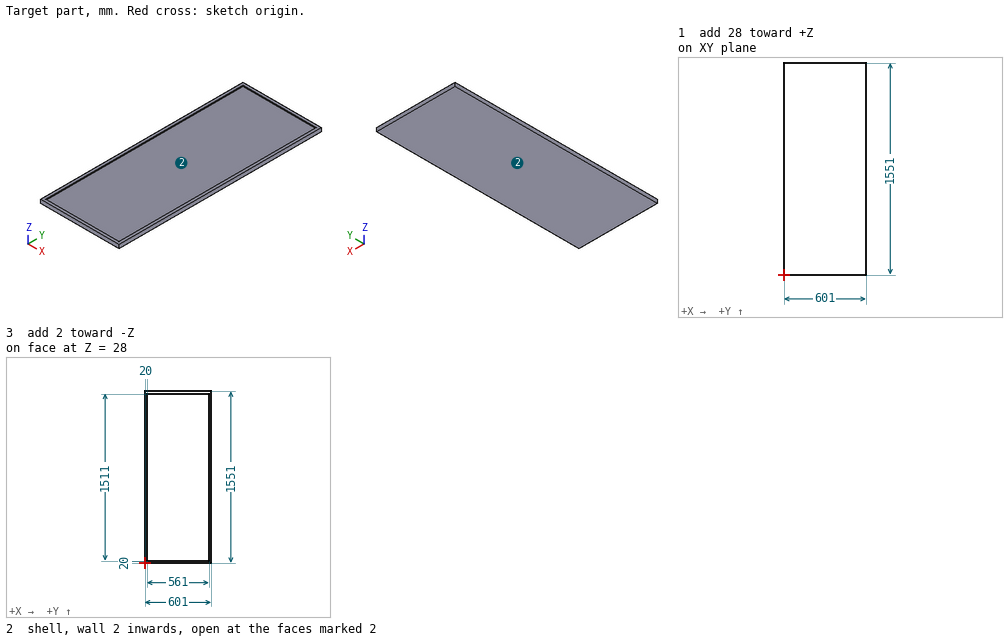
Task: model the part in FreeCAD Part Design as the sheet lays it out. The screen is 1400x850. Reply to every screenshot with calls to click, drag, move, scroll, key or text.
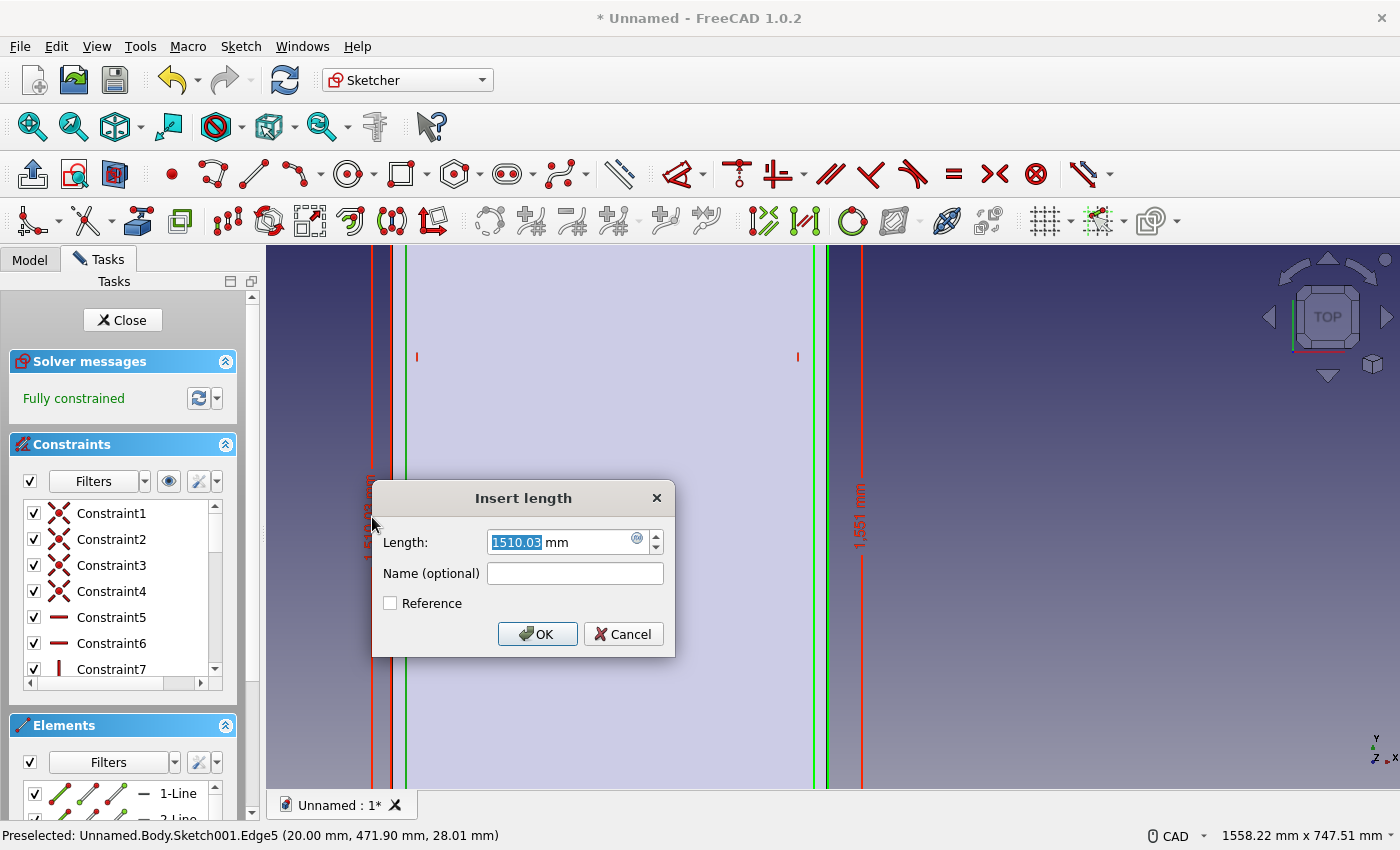
text(1511)
key(Return)
key(Escape)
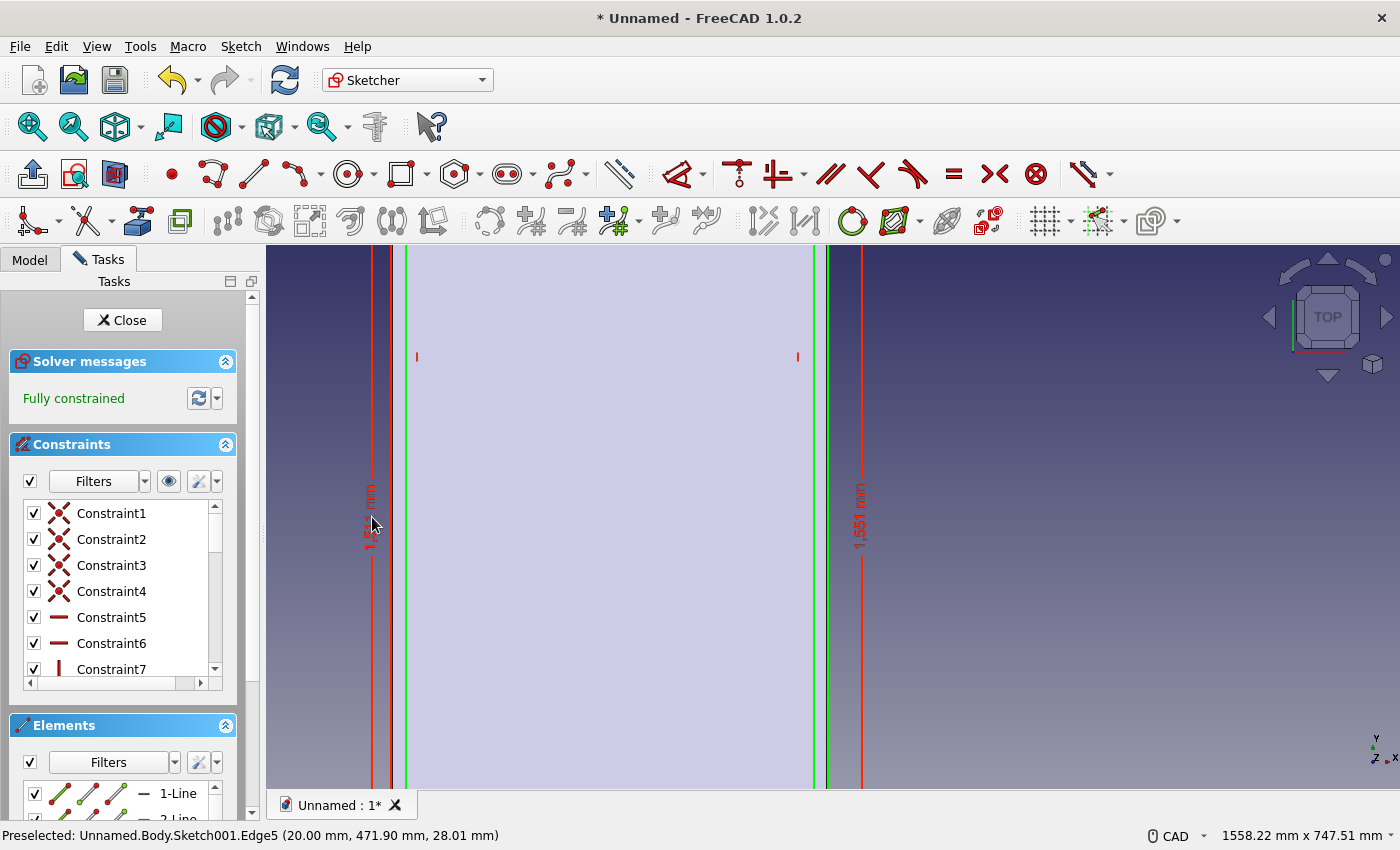
click(123, 320)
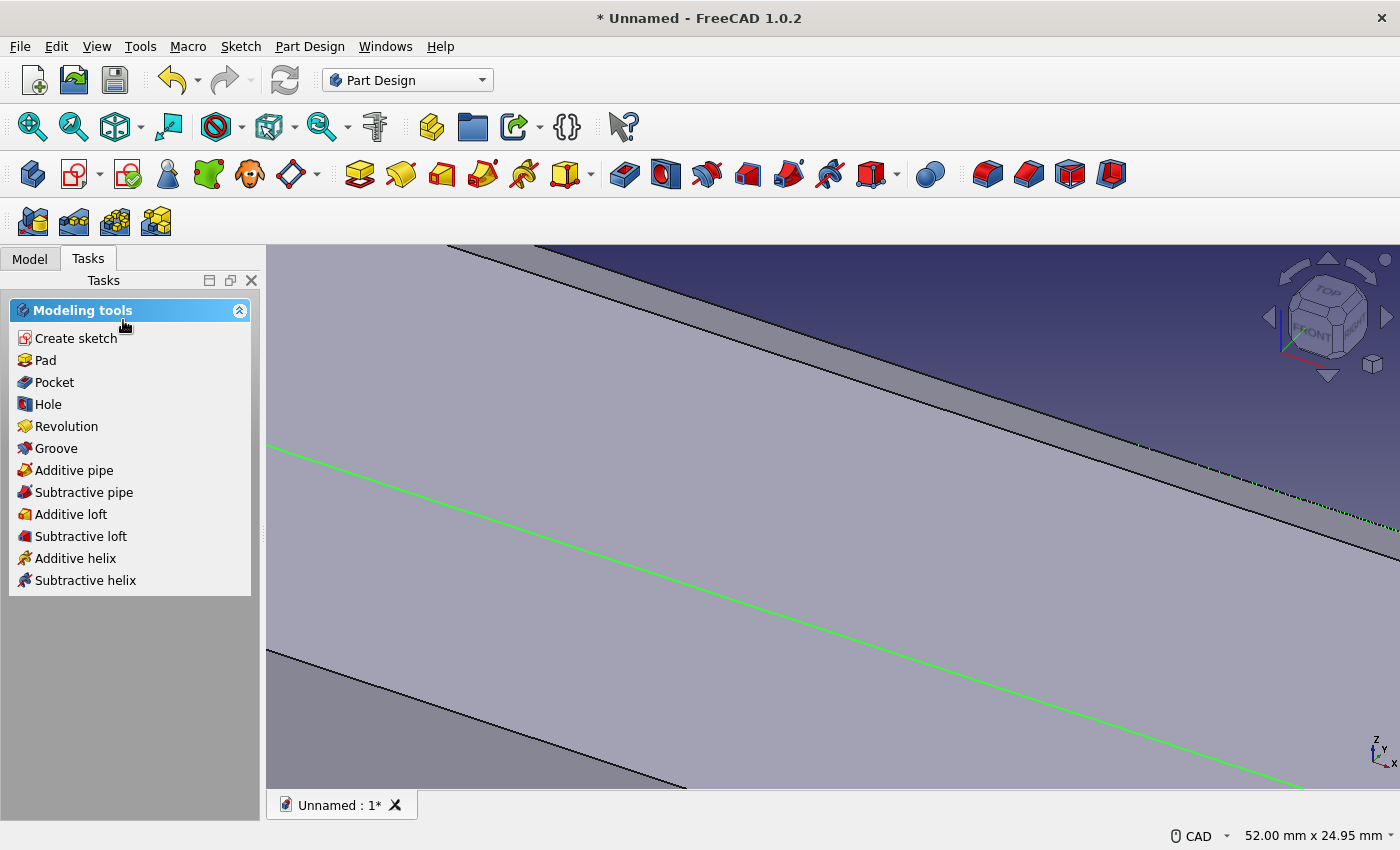
click(360, 174)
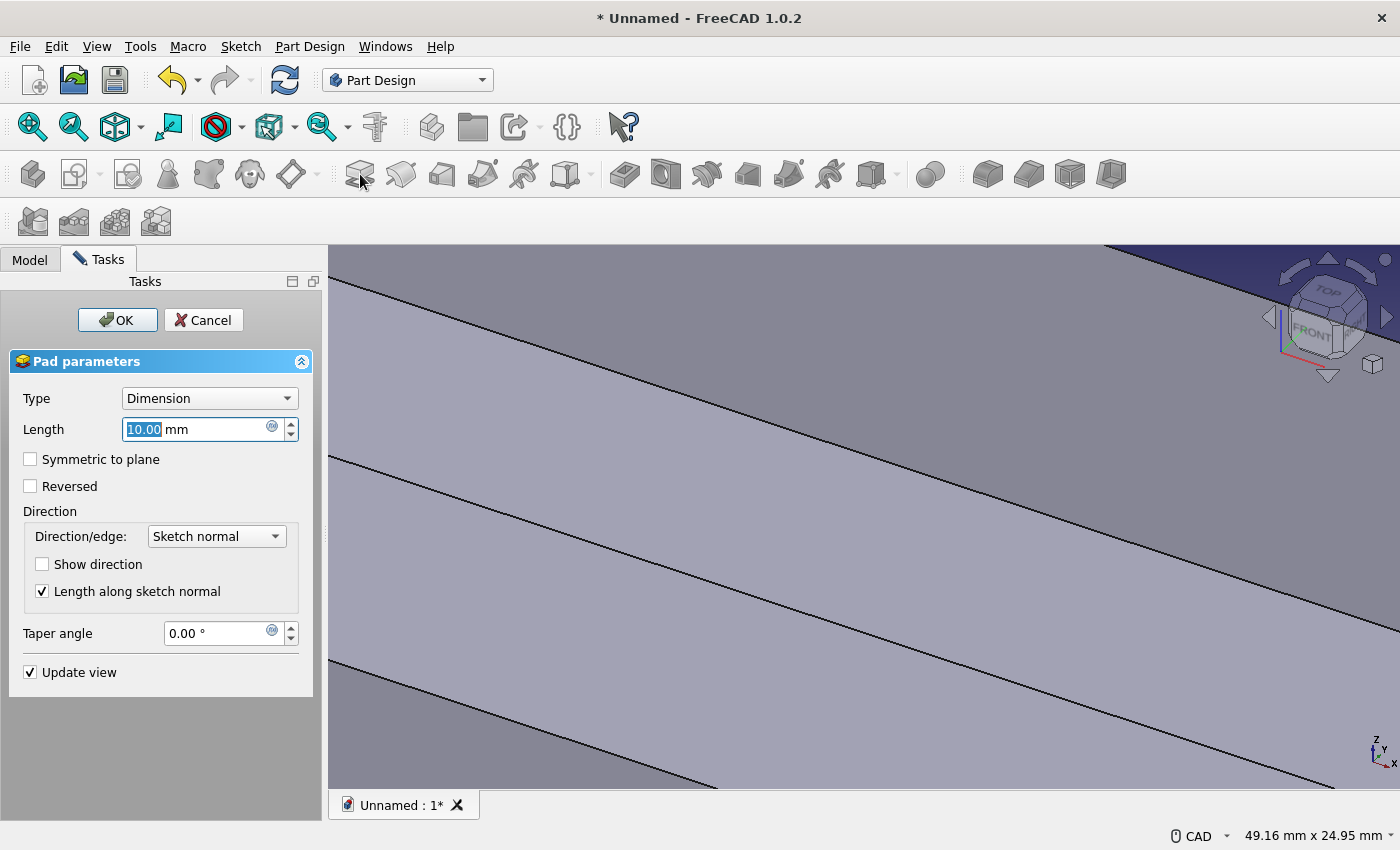
text(2)
key(Tab)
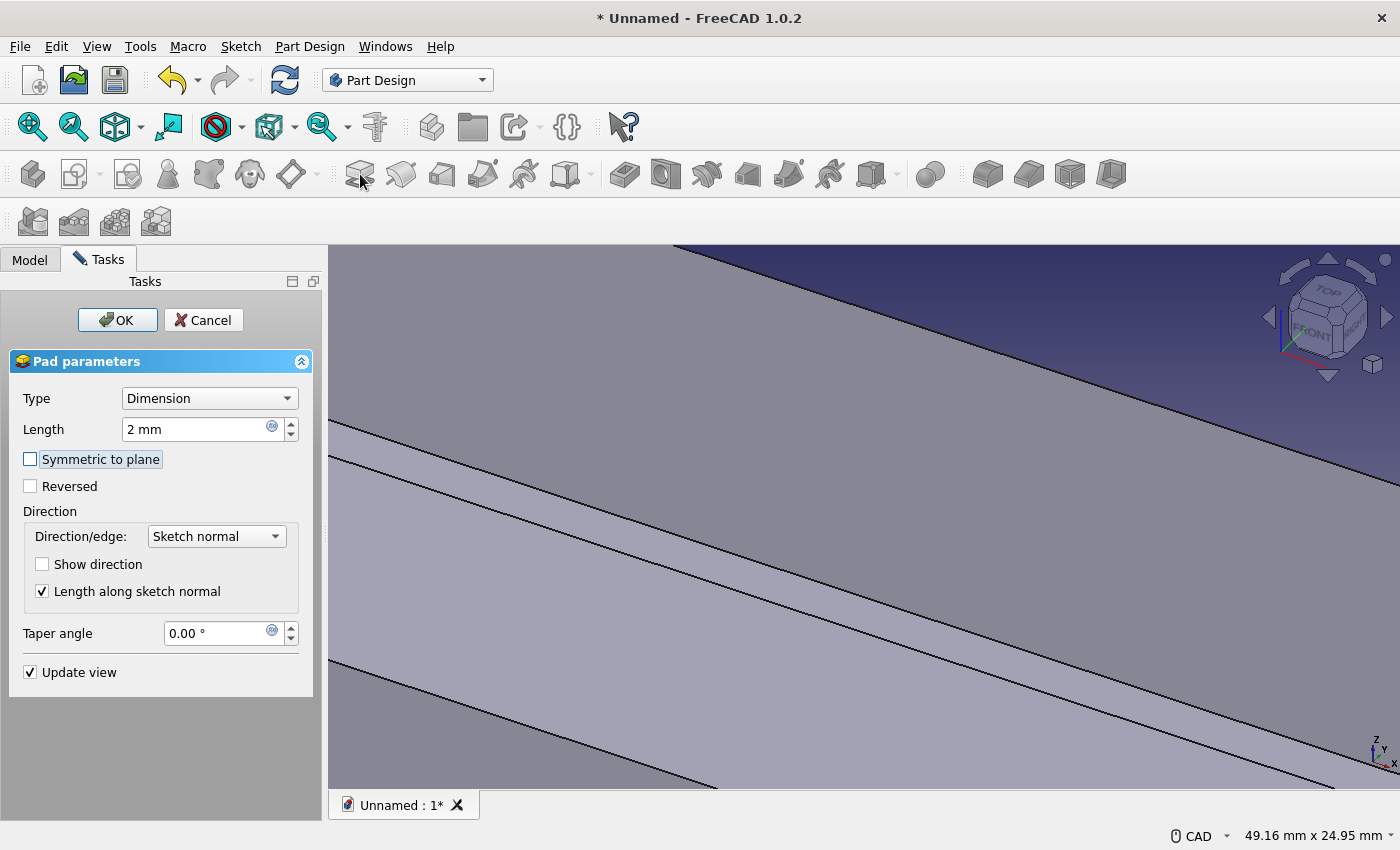
click(31, 486)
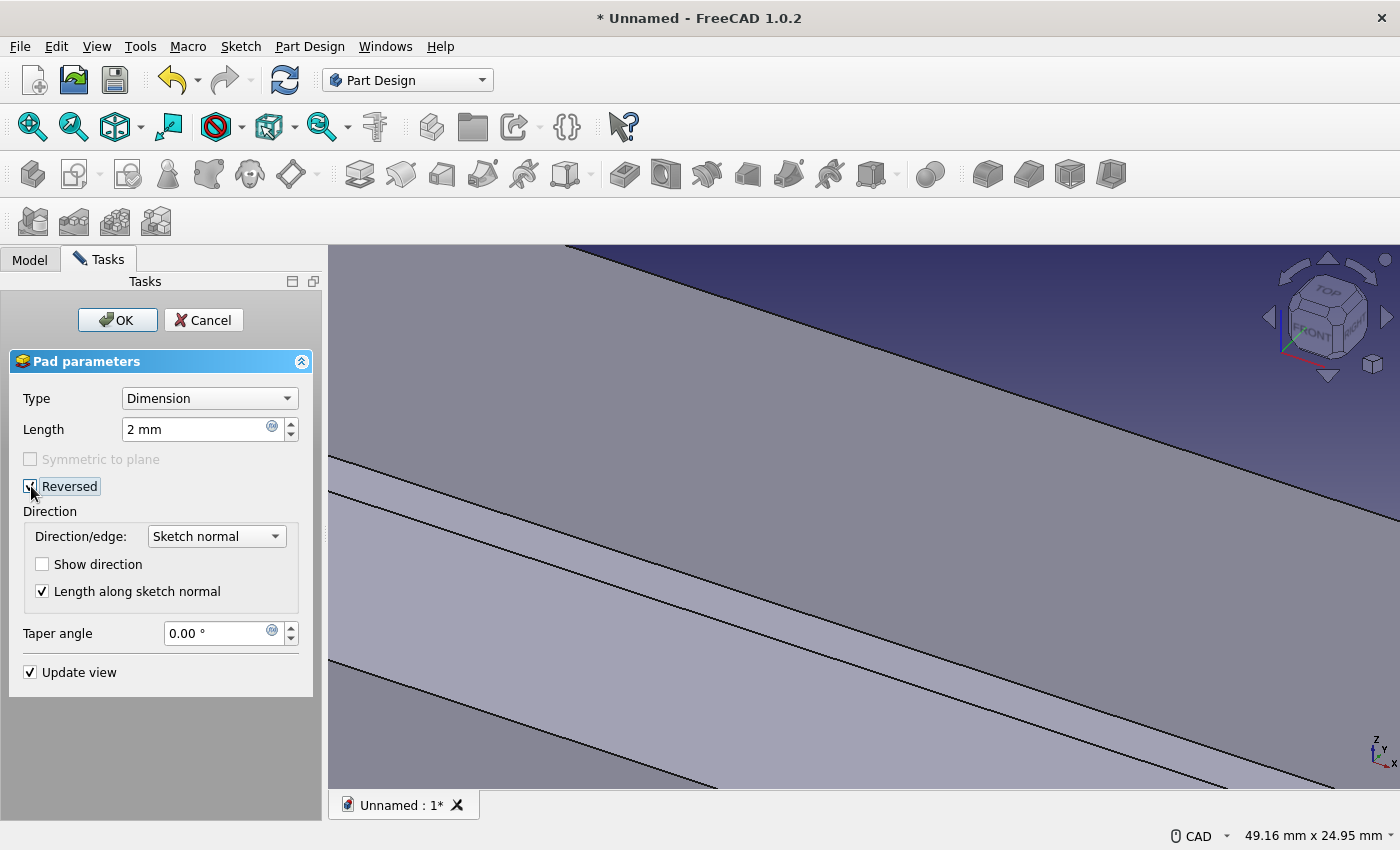
click(118, 320)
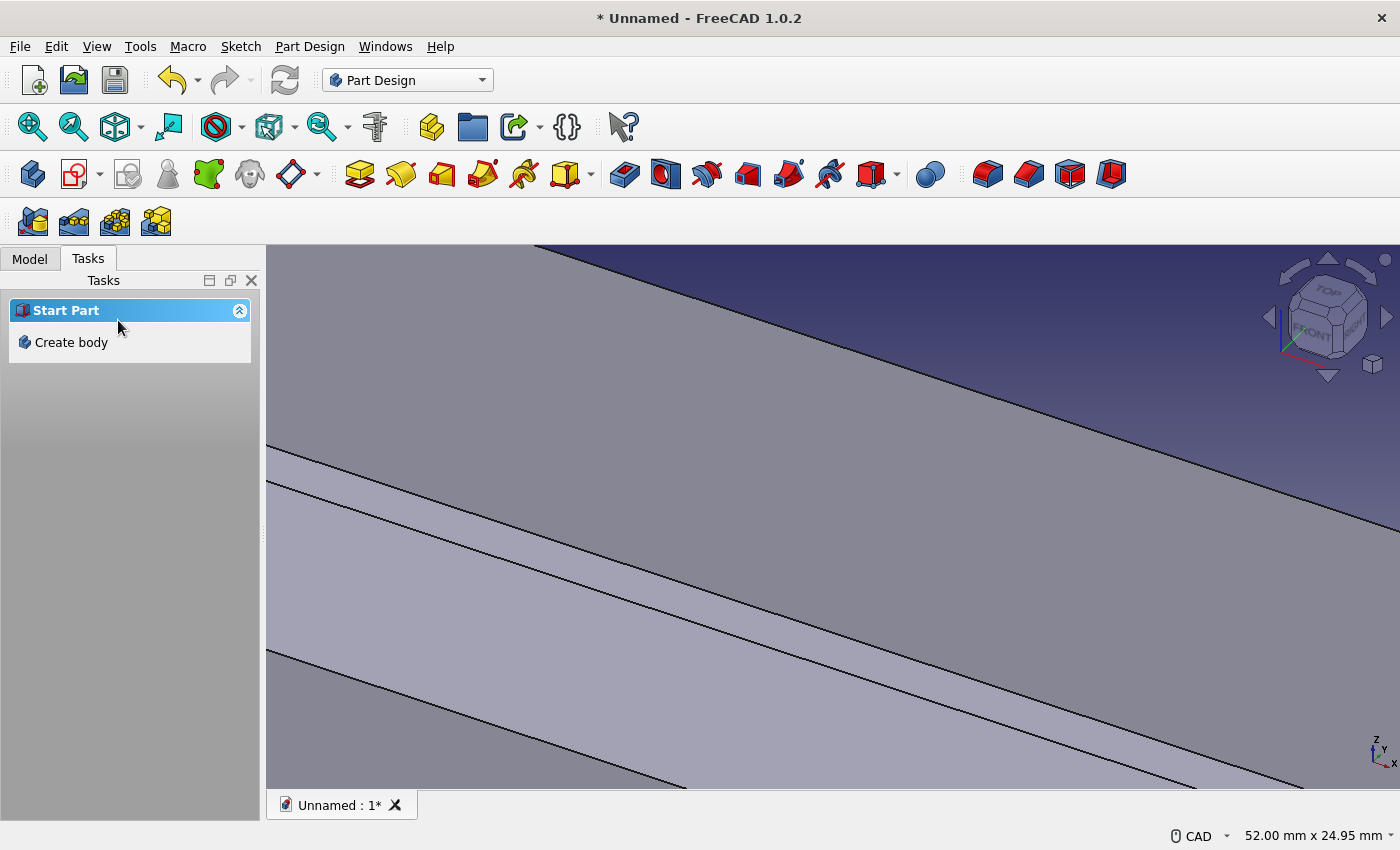
key(0)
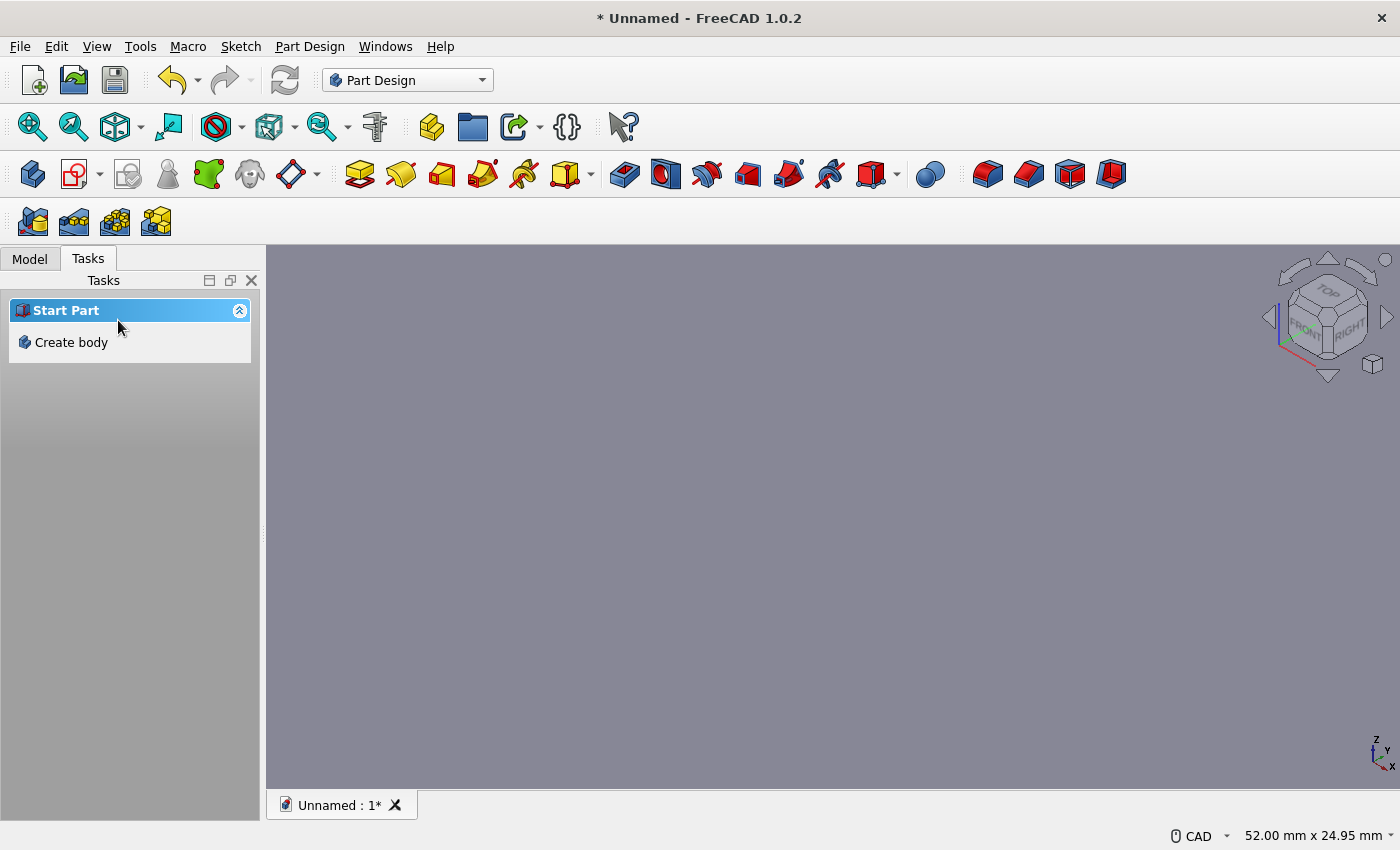
click(33, 128)